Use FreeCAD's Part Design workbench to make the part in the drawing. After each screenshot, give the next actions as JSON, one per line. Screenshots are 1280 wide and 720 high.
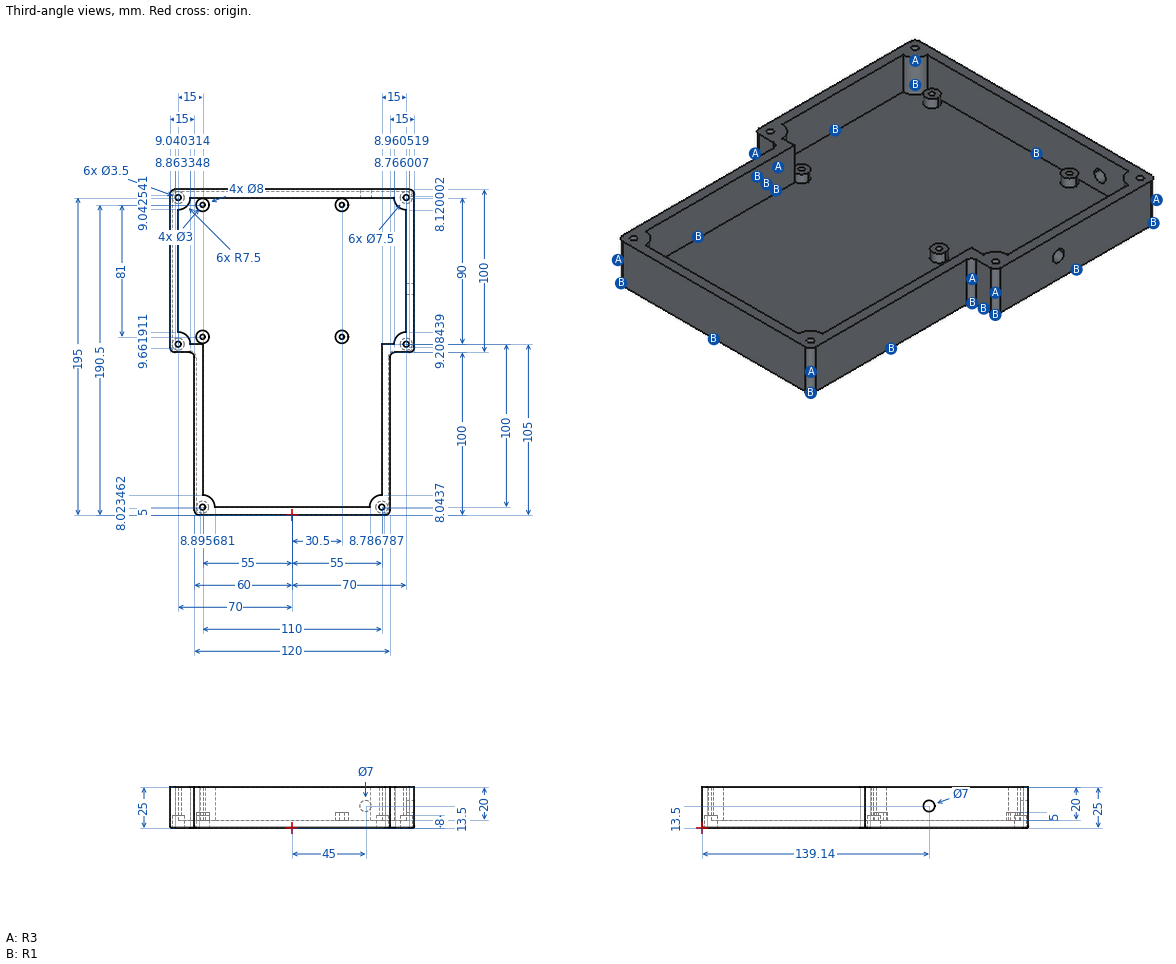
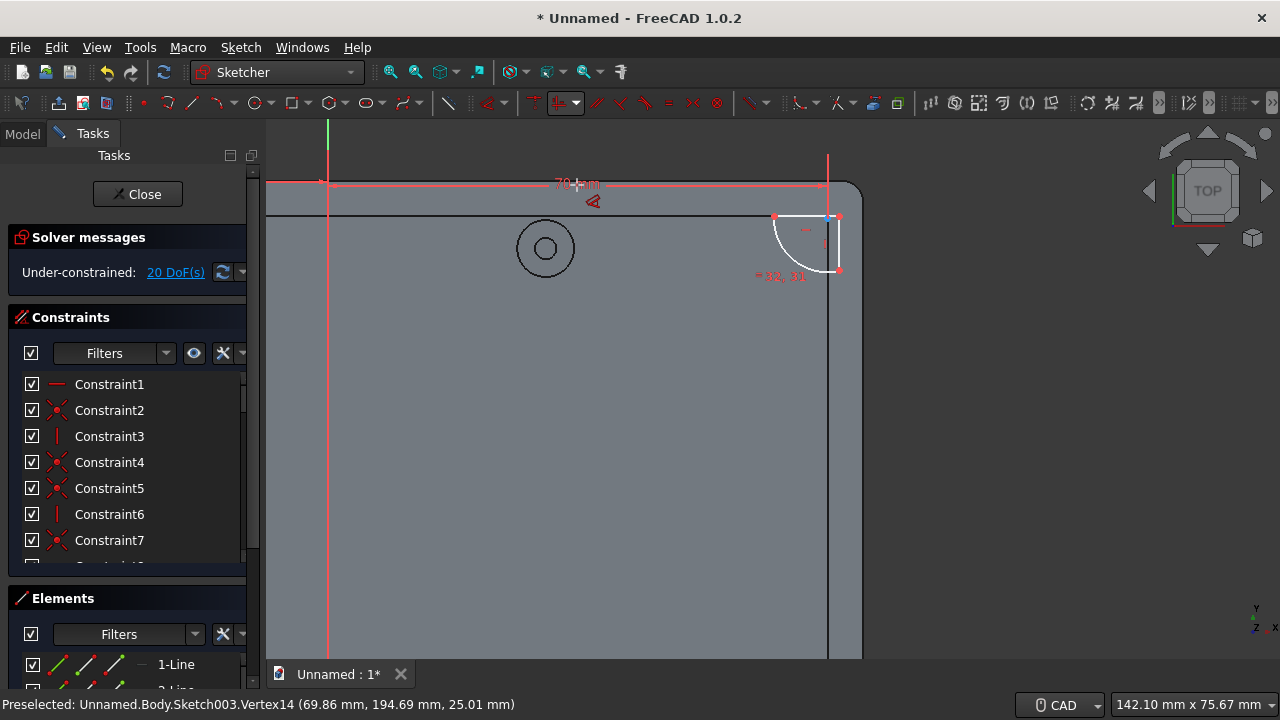
{"action": "scroll", "coordinate": [828, 220], "scroll_direction": "down", "scroll_amount": 7}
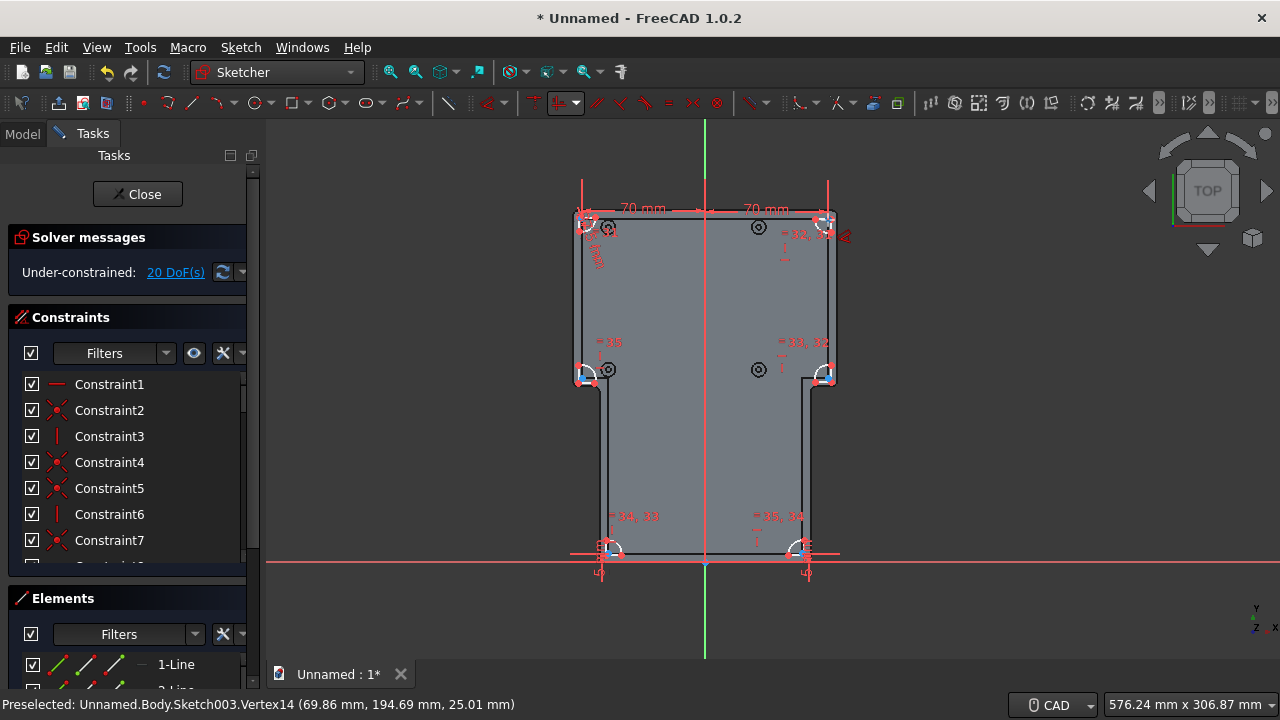
{"action": "scroll", "coordinate": [828, 378], "scroll_direction": "up", "scroll_amount": 5}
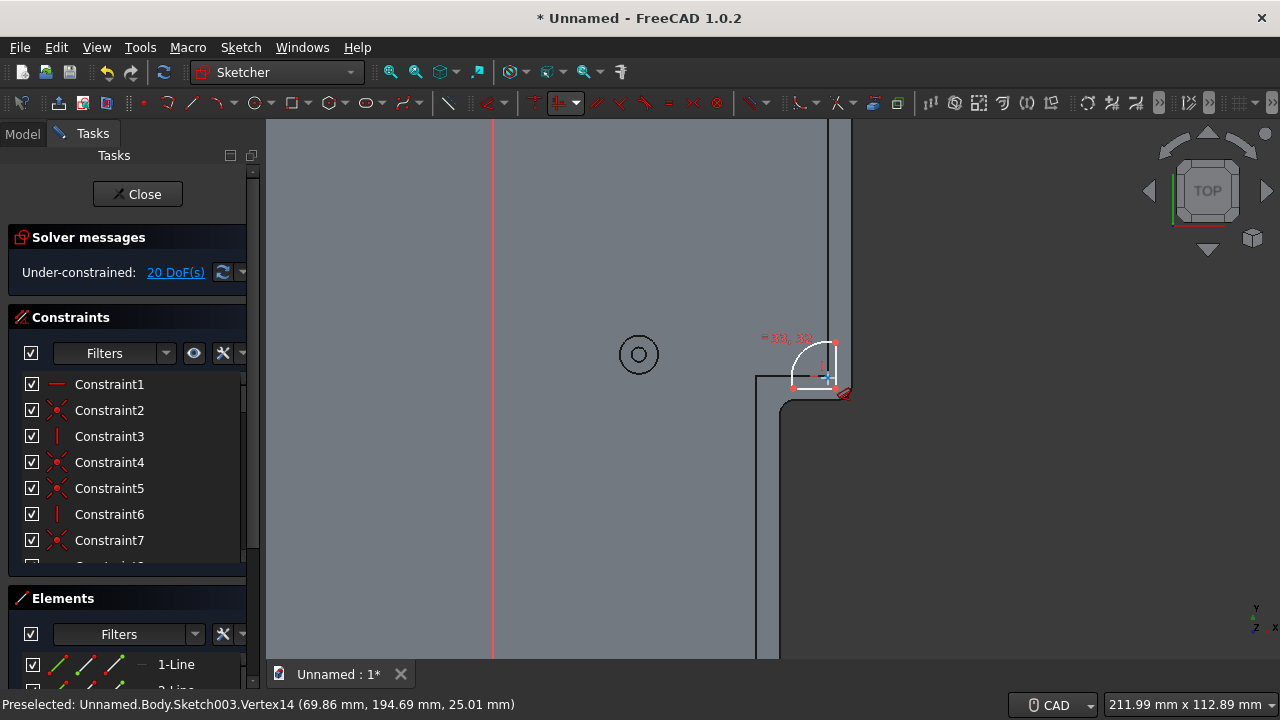
{"action": "left_click", "coordinate": [828, 378]}
{"action": "left_click", "coordinate": [660, 344]}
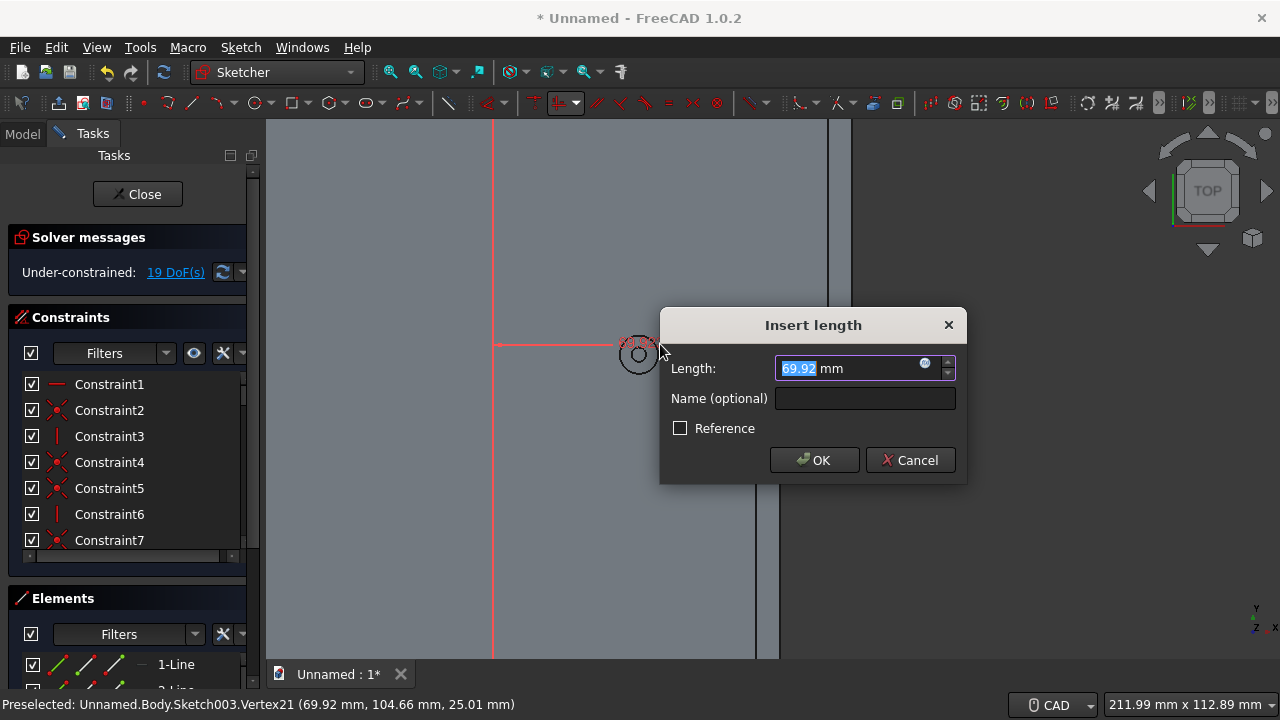
{"action": "type", "text": "70"}
{"action": "key", "text": "Return"}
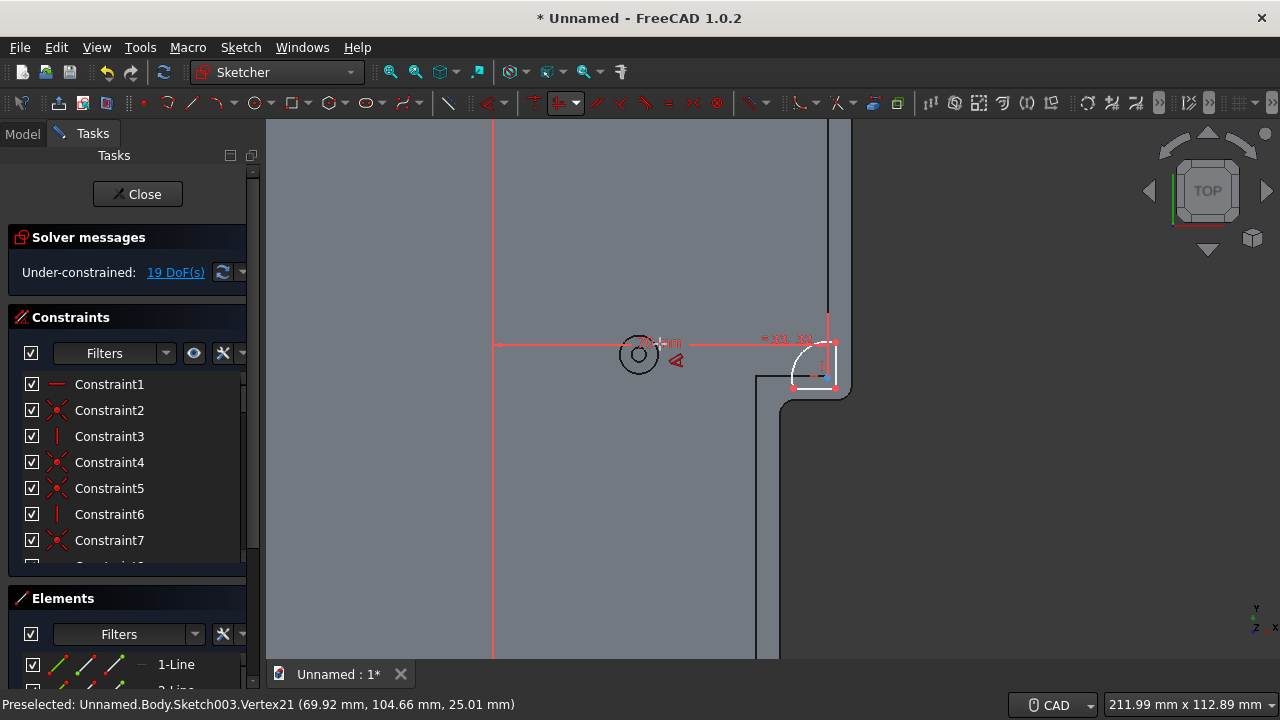
{"action": "scroll", "coordinate": [828, 378], "scroll_direction": "down", "scroll_amount": 5}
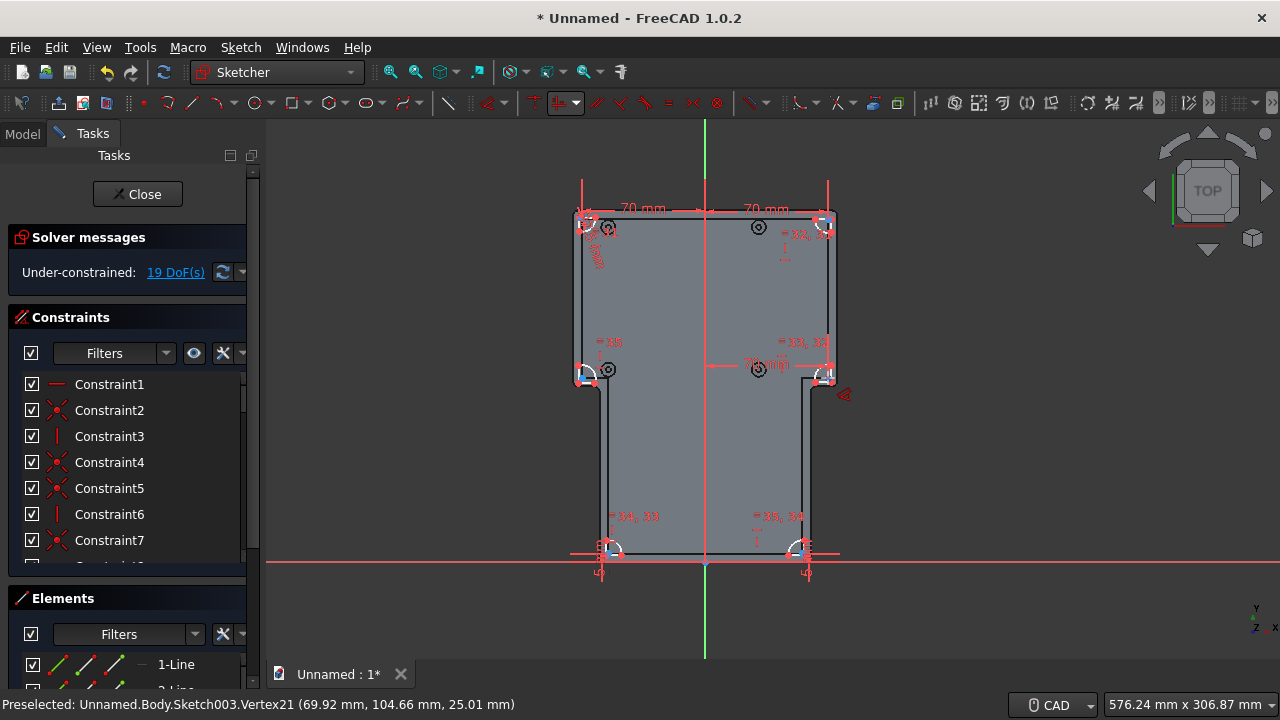
{"action": "scroll", "coordinate": [608, 554], "scroll_direction": "up", "scroll_amount": 8}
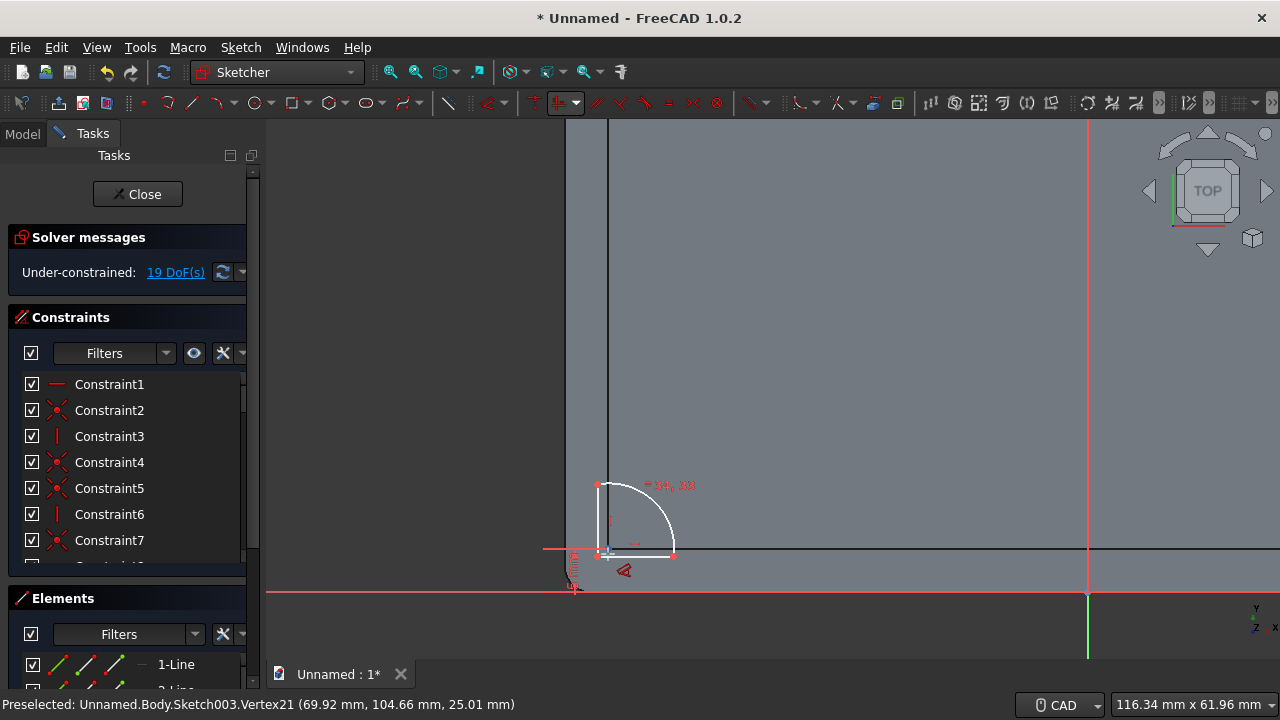
{"action": "left_click", "coordinate": [609, 549]}
{"action": "left_click", "coordinate": [848, 626]}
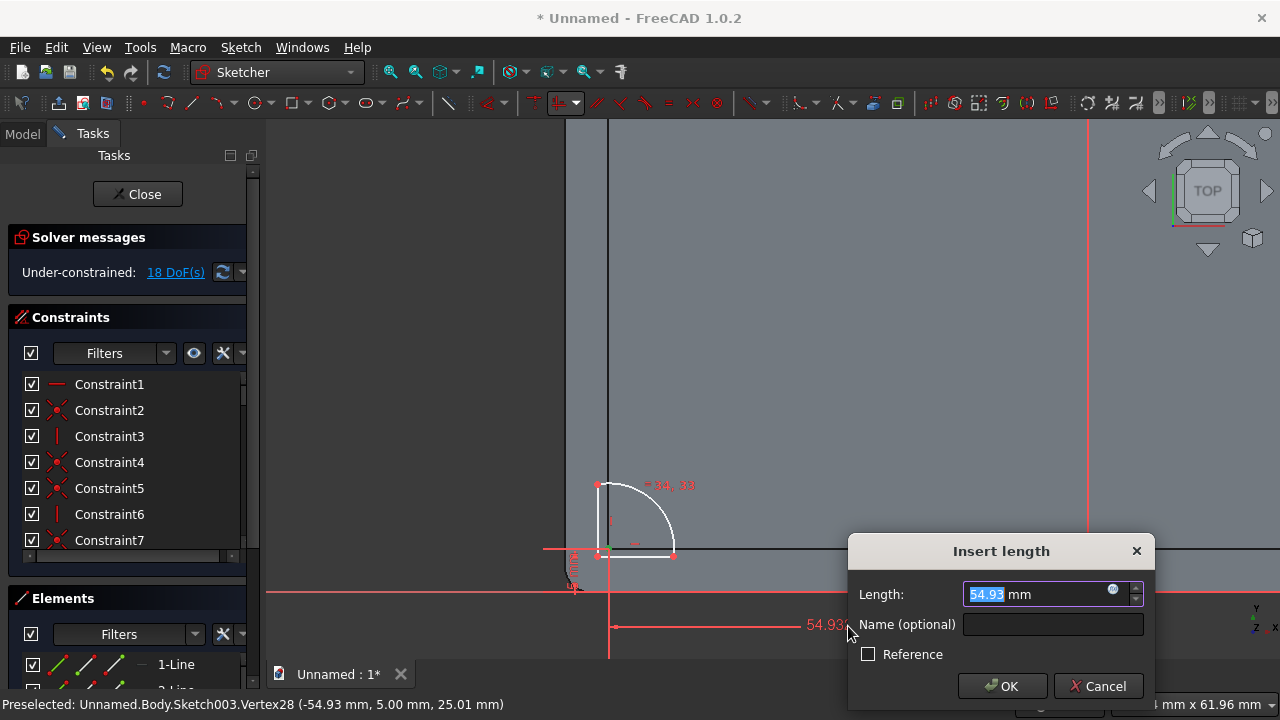
{"action": "type", "text": "55"}
{"action": "key", "text": "Return"}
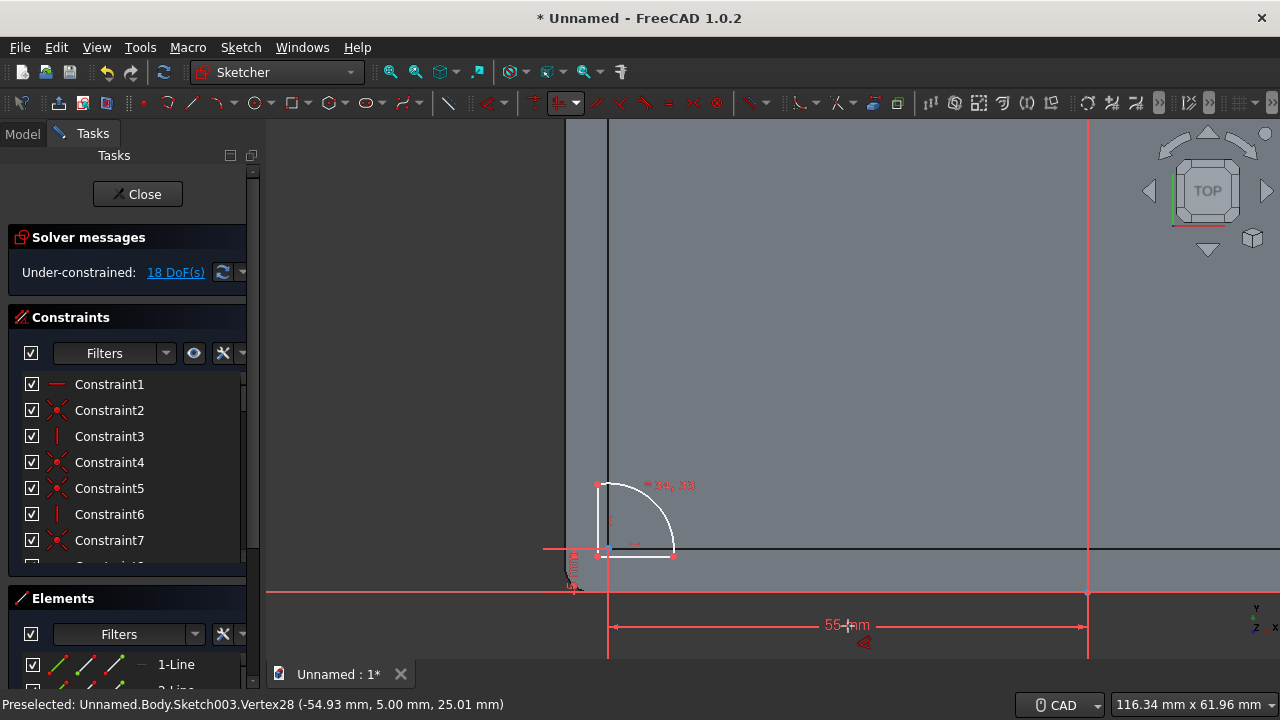
{"action": "scroll", "coordinate": [608, 554], "scroll_direction": "down", "scroll_amount": 8}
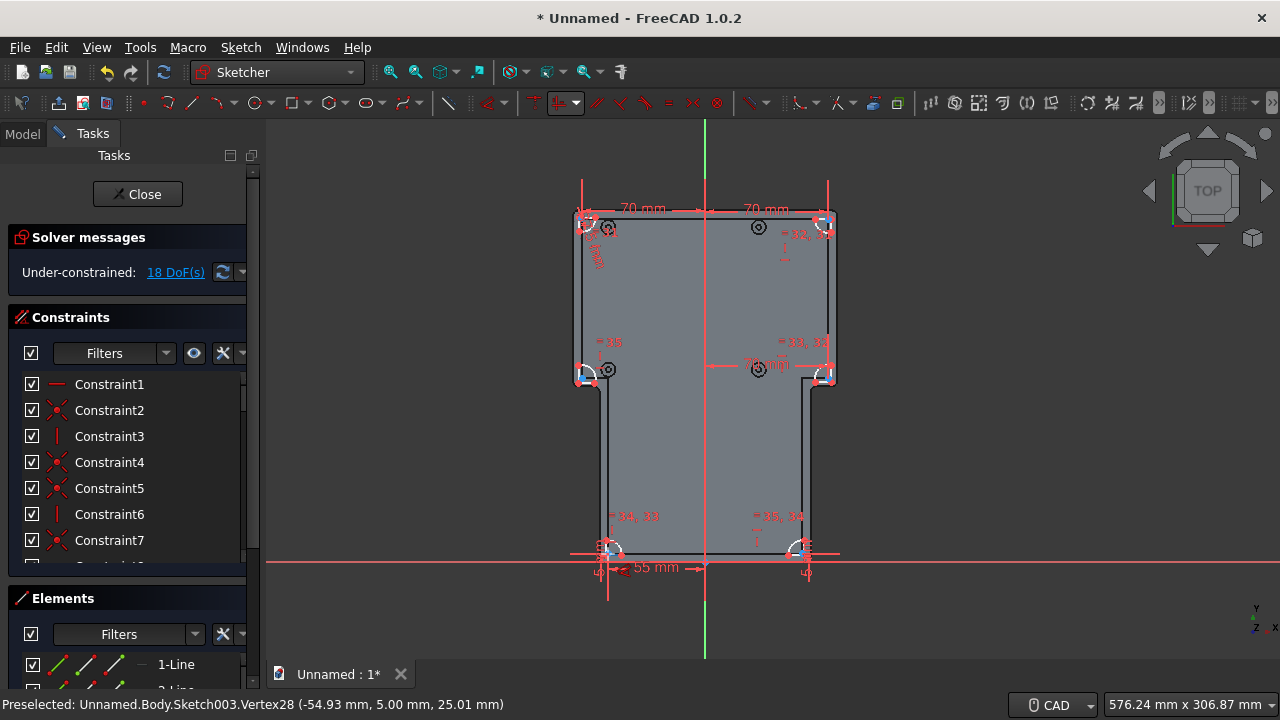
{"action": "scroll", "coordinate": [802, 554], "scroll_direction": "up", "scroll_amount": 8}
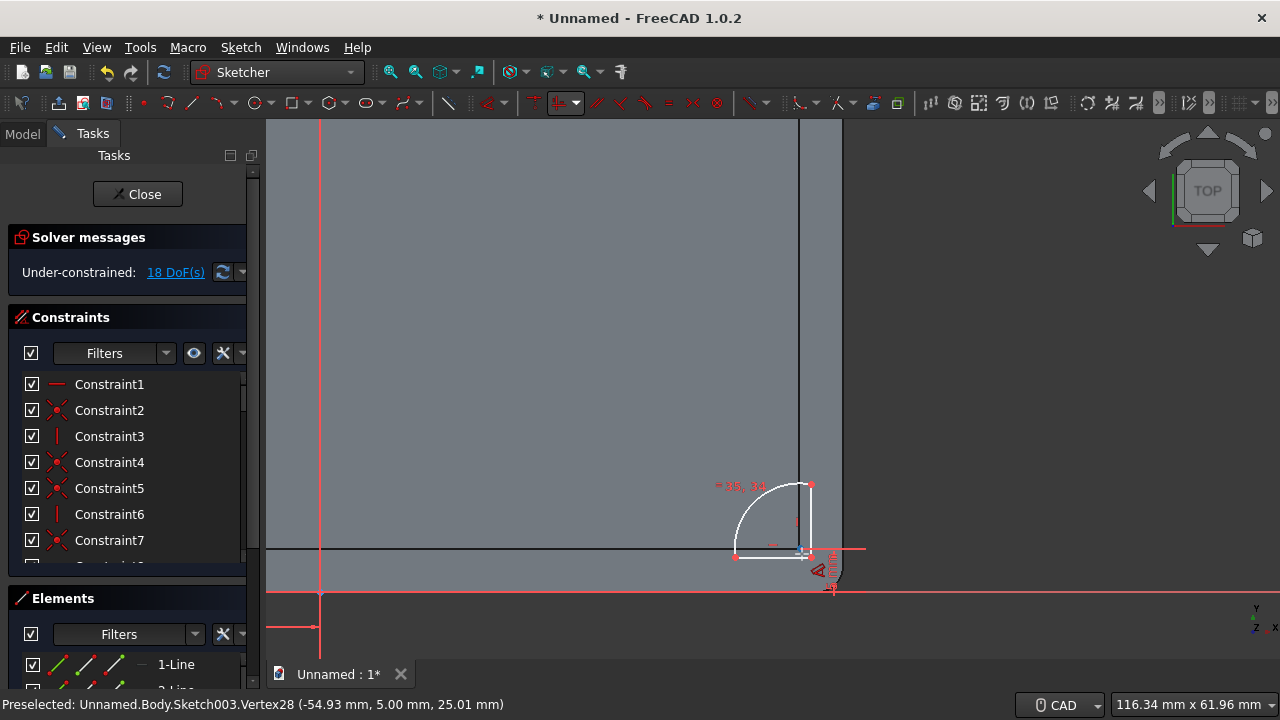
{"action": "left_click", "coordinate": [800, 549]}
{"action": "left_click", "coordinate": [560, 626]}